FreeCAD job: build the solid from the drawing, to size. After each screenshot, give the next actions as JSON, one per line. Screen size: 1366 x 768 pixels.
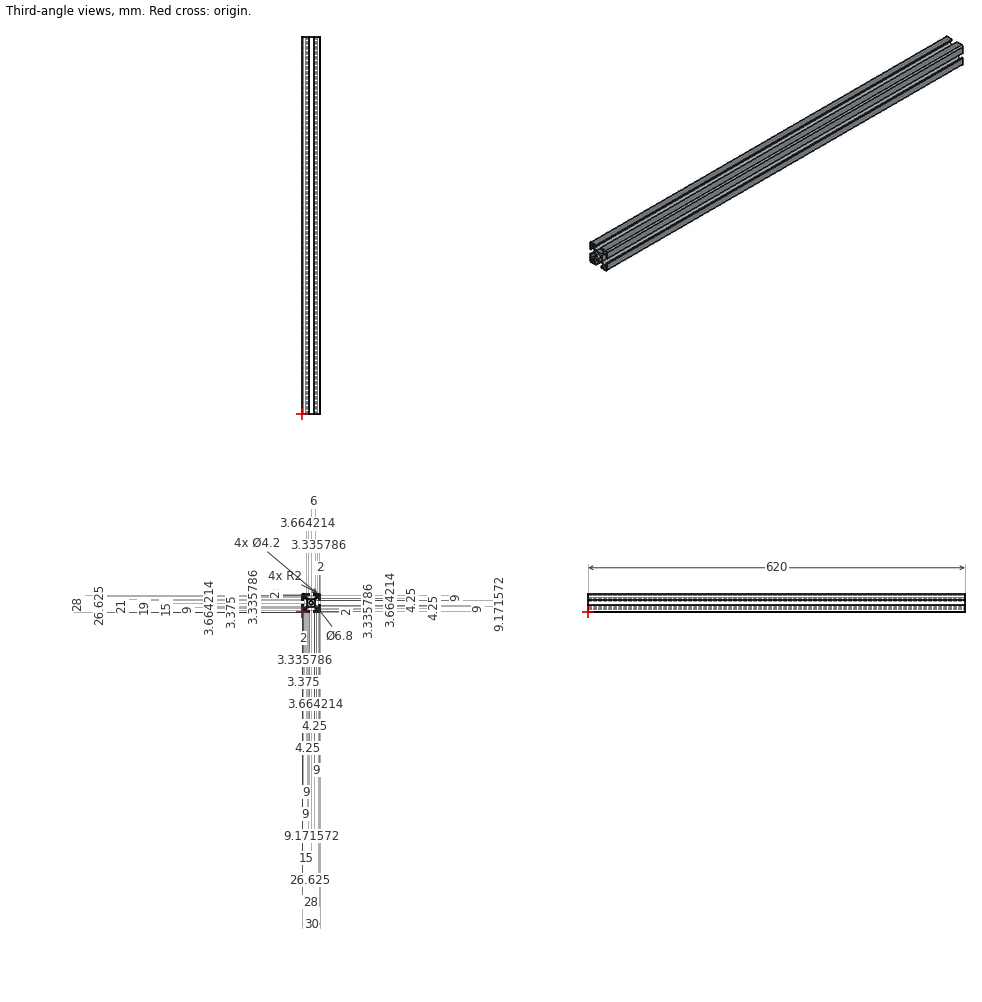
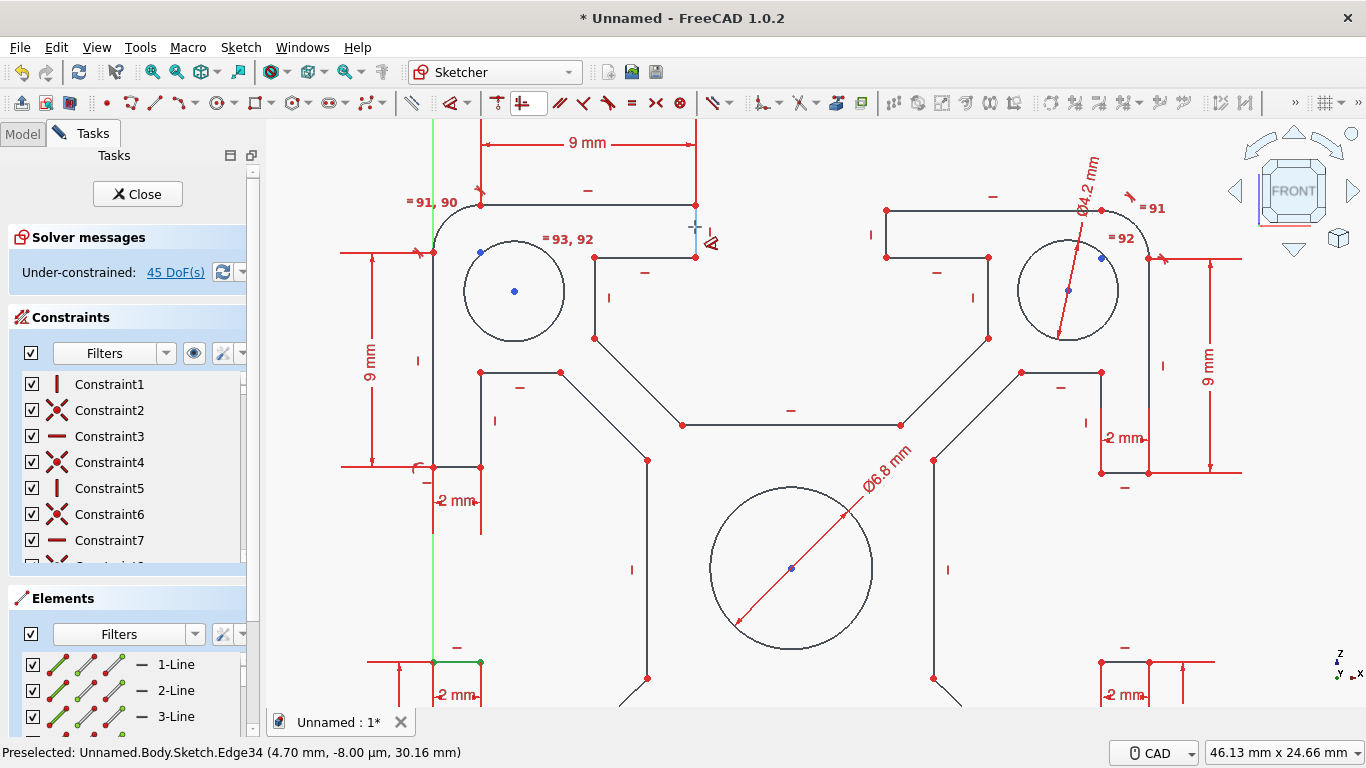
{"action": "left_click", "coordinate": [696, 226]}
{"action": "left_click", "coordinate": [662, 231]}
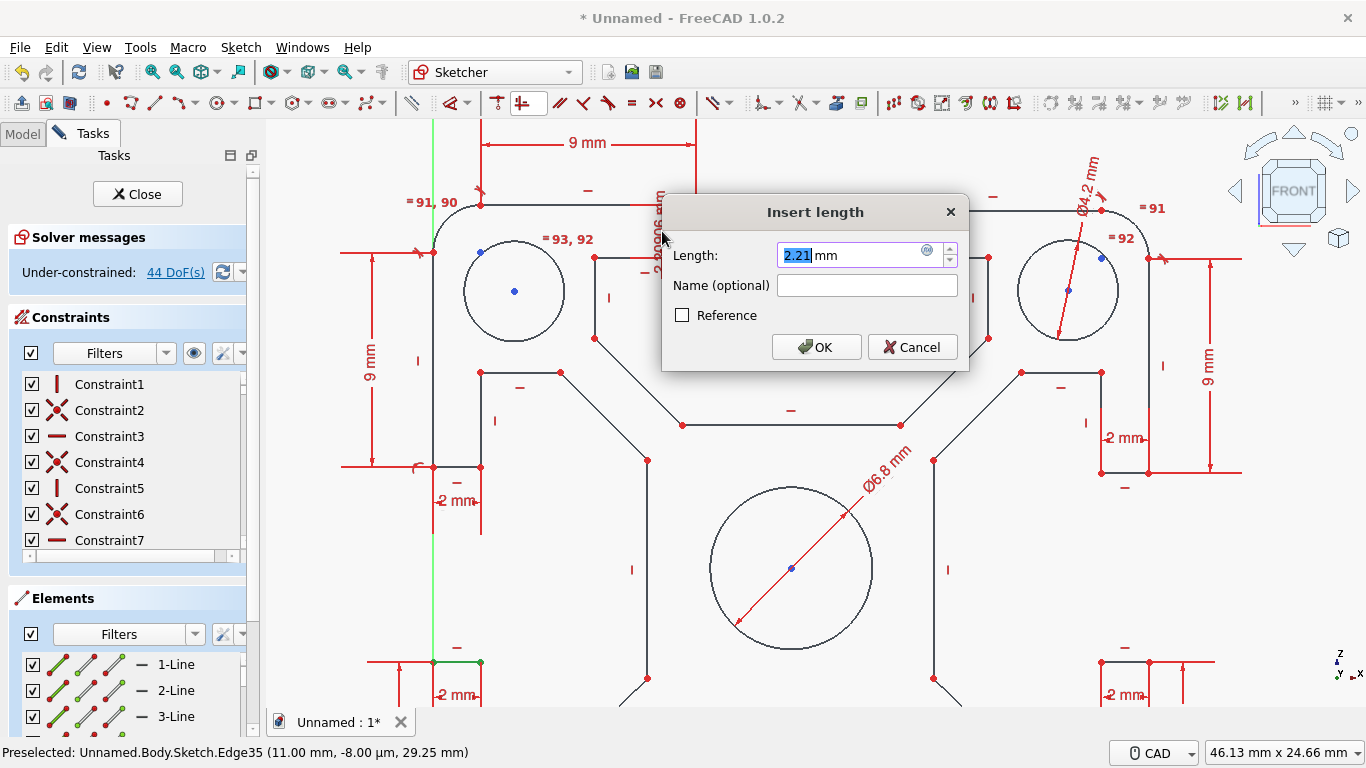
{"action": "type", "text": "2"}
{"action": "key", "text": "Return"}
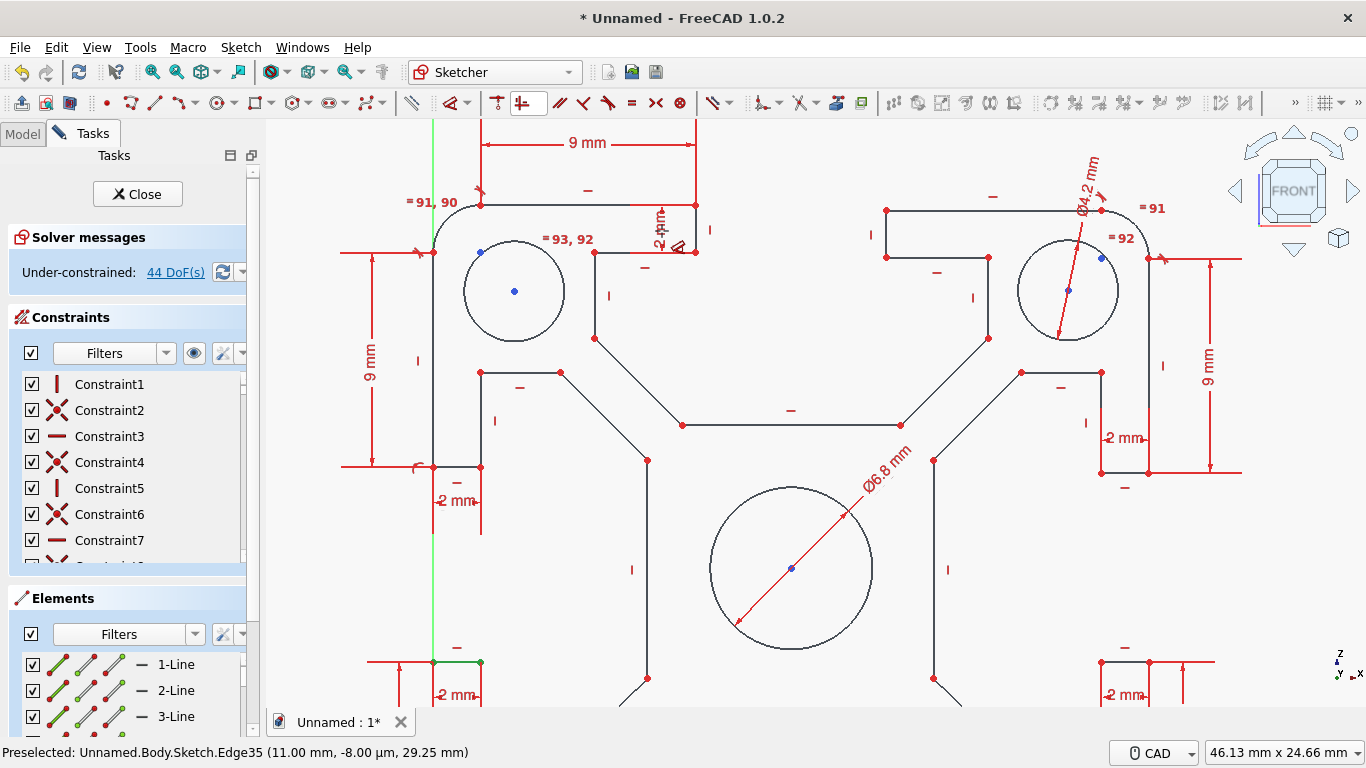
{"action": "left_click", "coordinate": [886, 244]}
{"action": "left_click", "coordinate": [920, 234]}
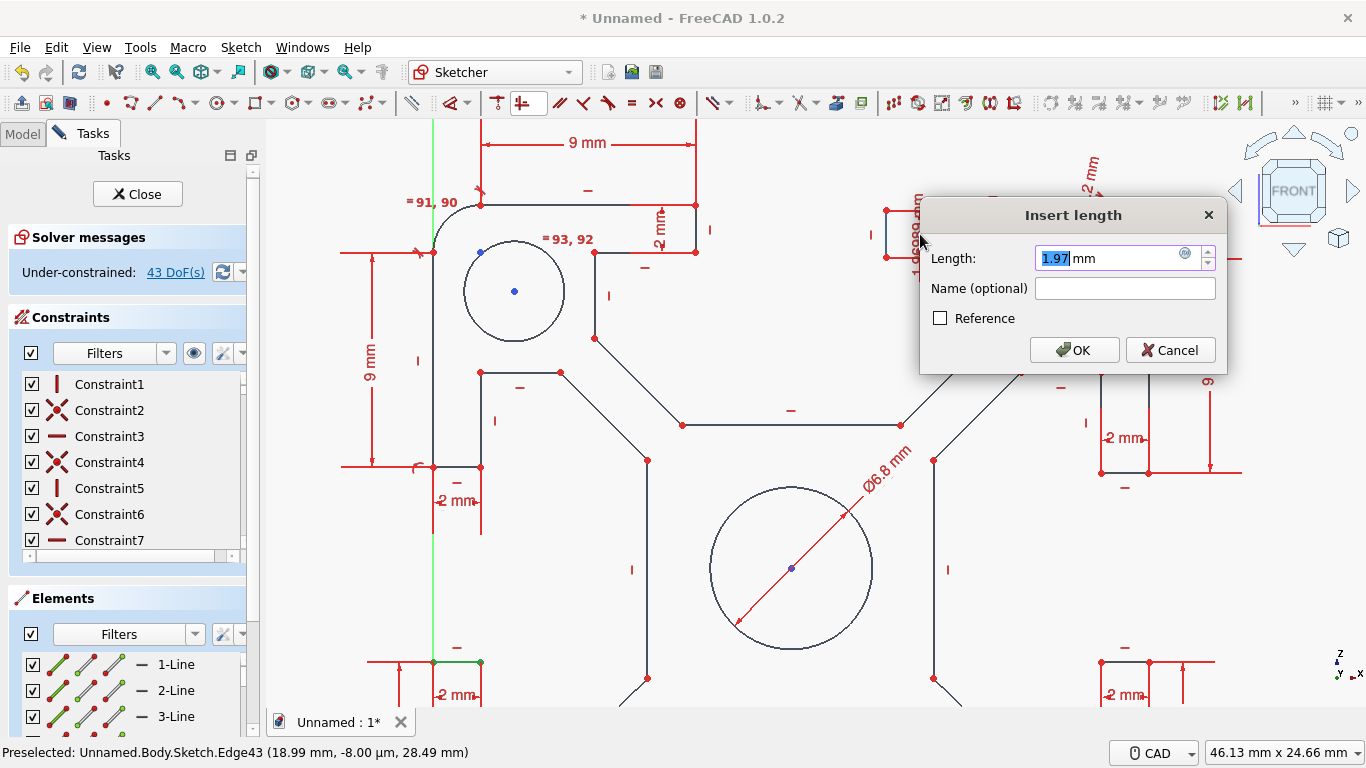
{"action": "type", "text": "2"}
{"action": "key", "text": "Return"}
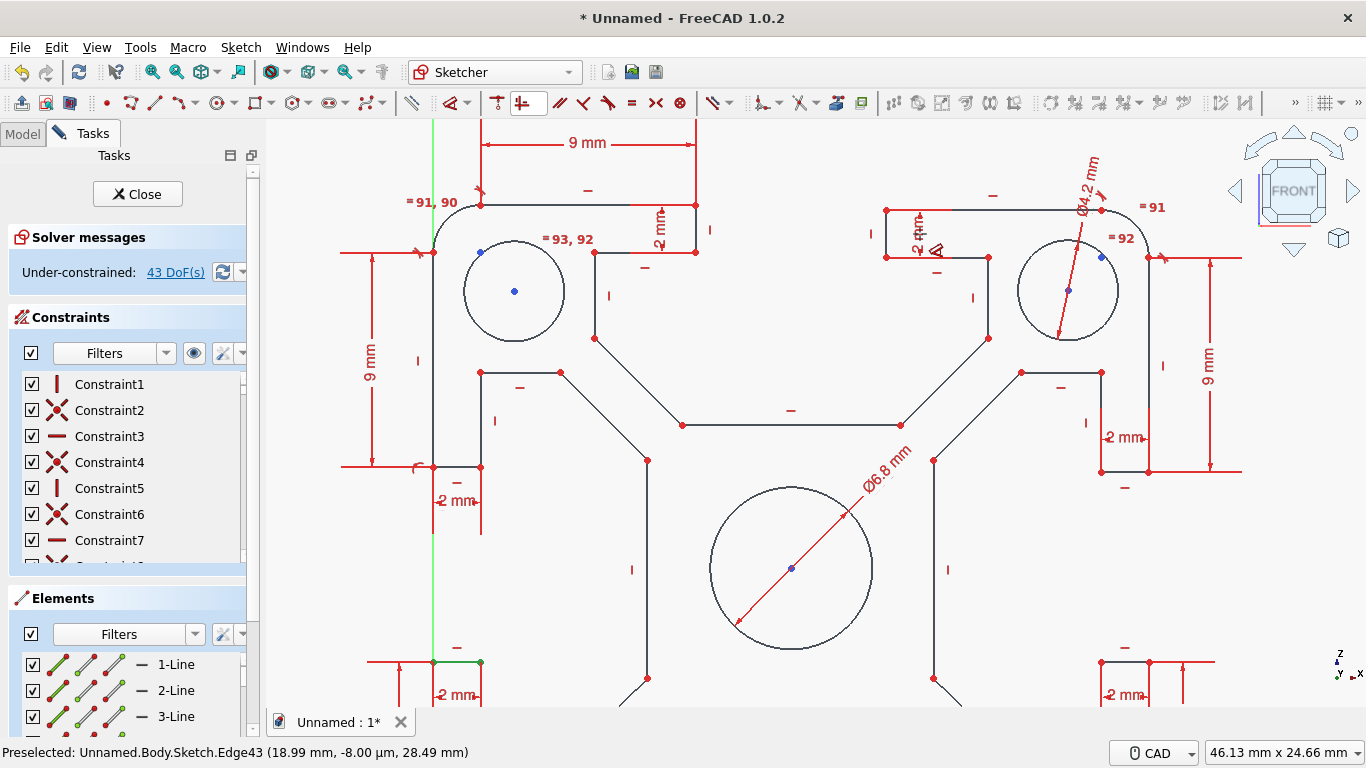
{"action": "left_click", "coordinate": [951, 210]}
{"action": "left_click", "coordinate": [994, 176]}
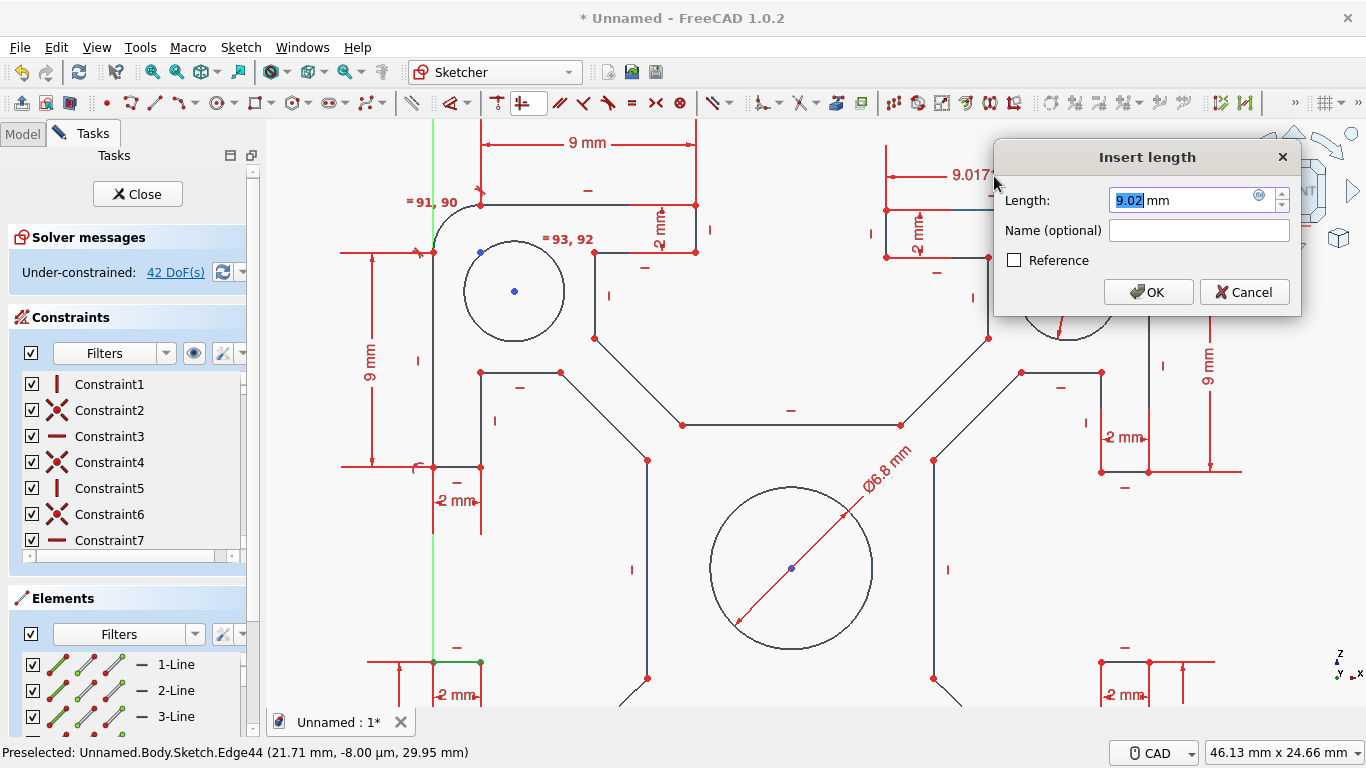
{"action": "type", "text": "9"}
{"action": "key", "text": "Return"}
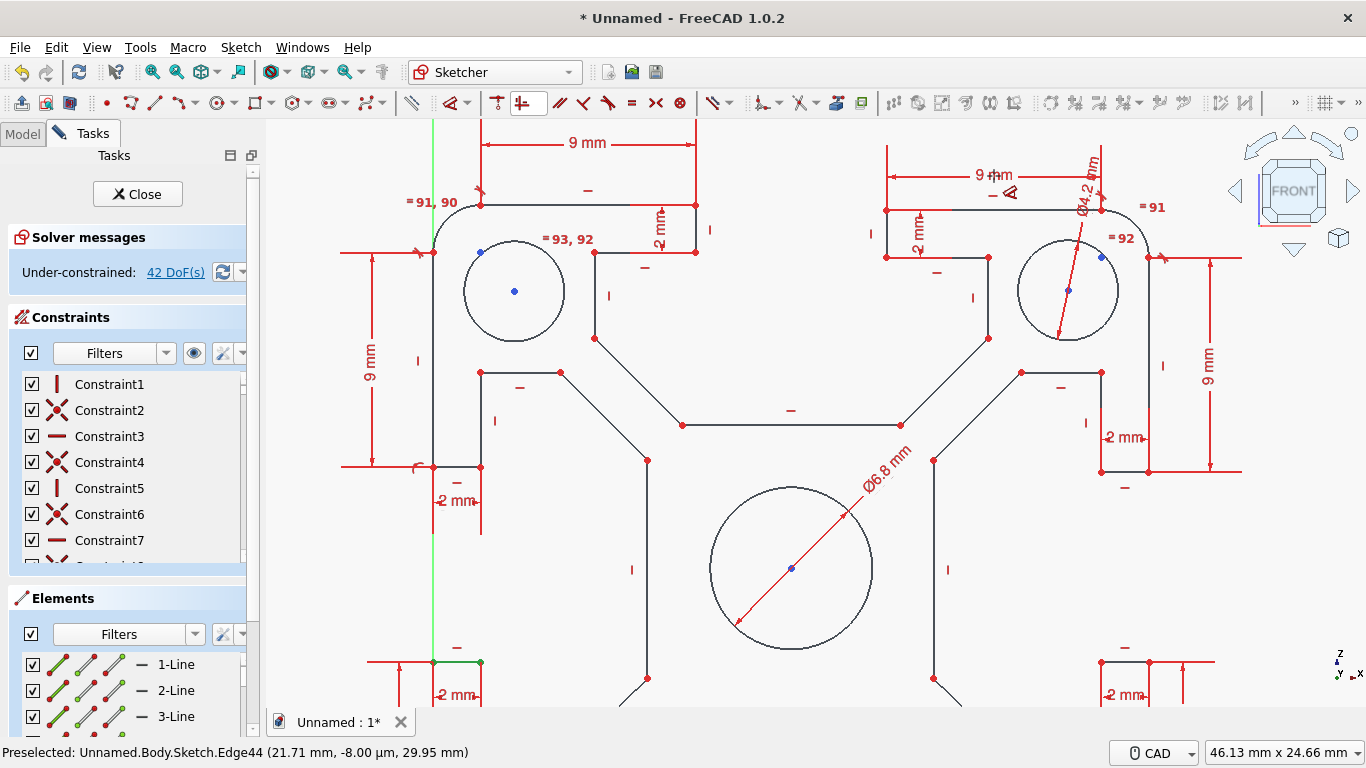
{"action": "scroll", "coordinate": [695, 226], "scroll_direction": "down", "scroll_amount": 3}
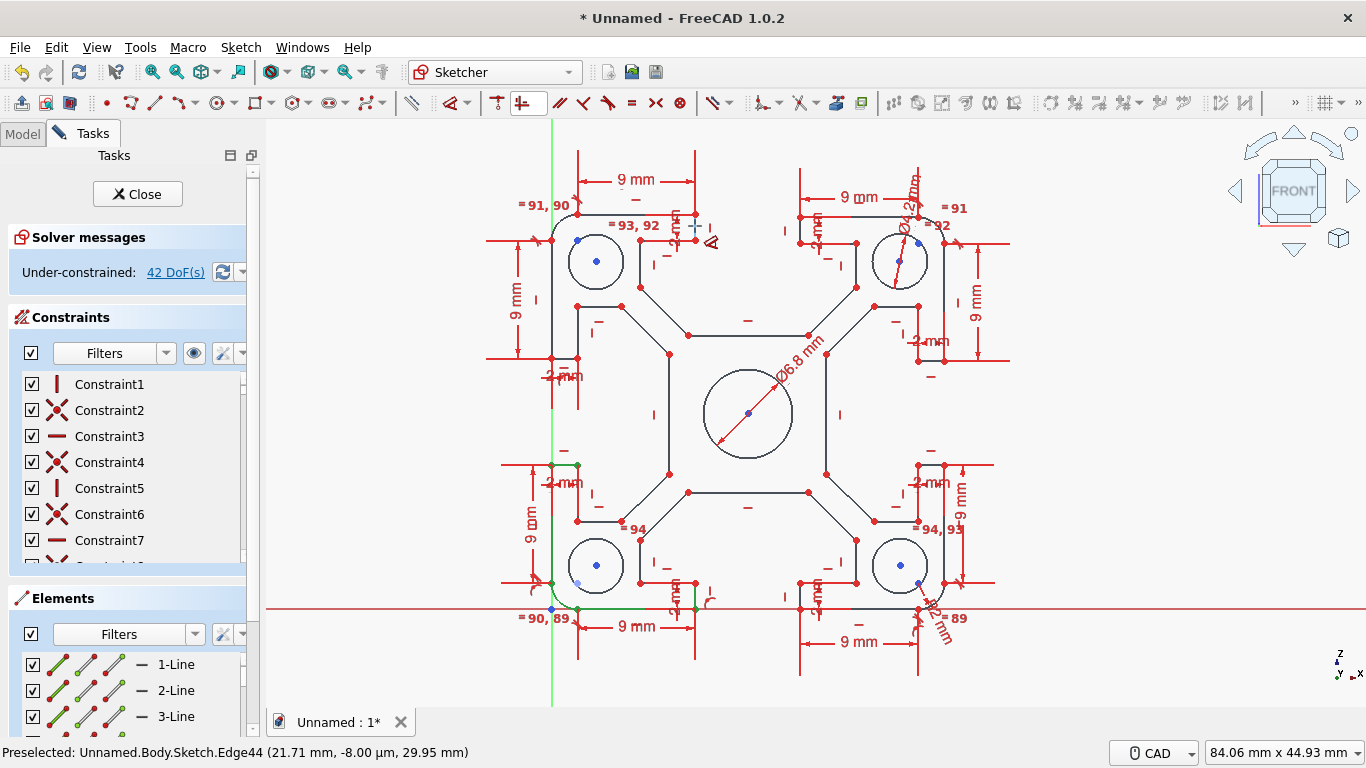
{"action": "left_click", "coordinate": [808, 493]}
{"action": "left_click", "coordinate": [518, 551]}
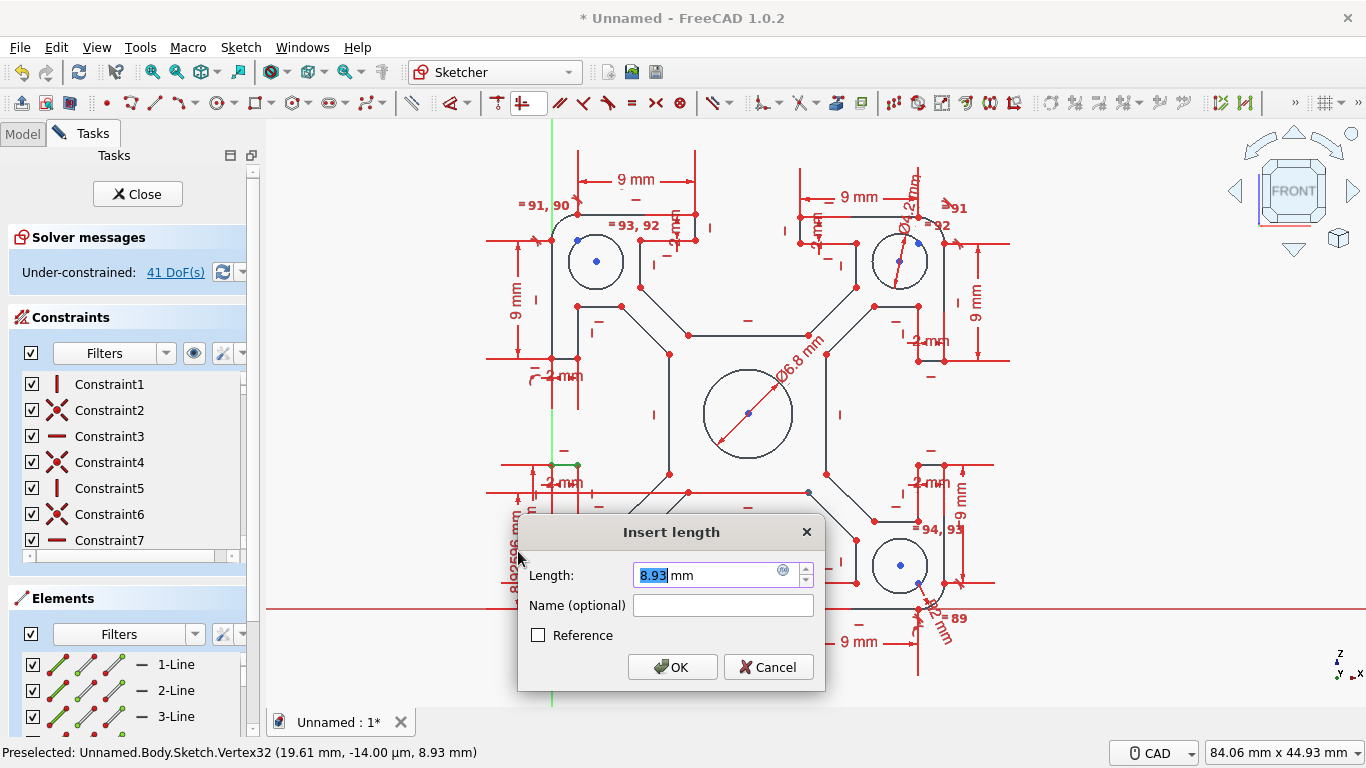
{"action": "type", "text": "9"}
{"action": "key", "text": "Return"}